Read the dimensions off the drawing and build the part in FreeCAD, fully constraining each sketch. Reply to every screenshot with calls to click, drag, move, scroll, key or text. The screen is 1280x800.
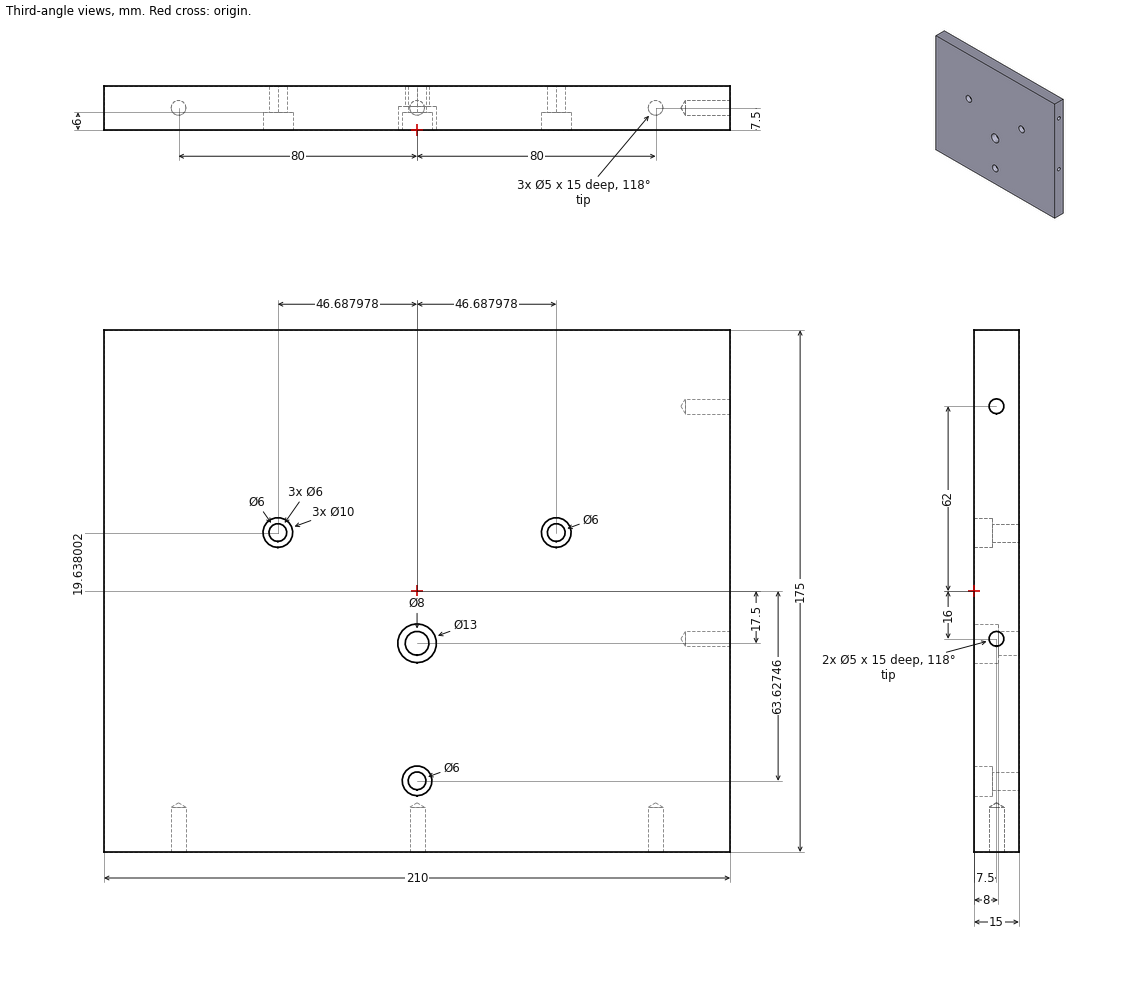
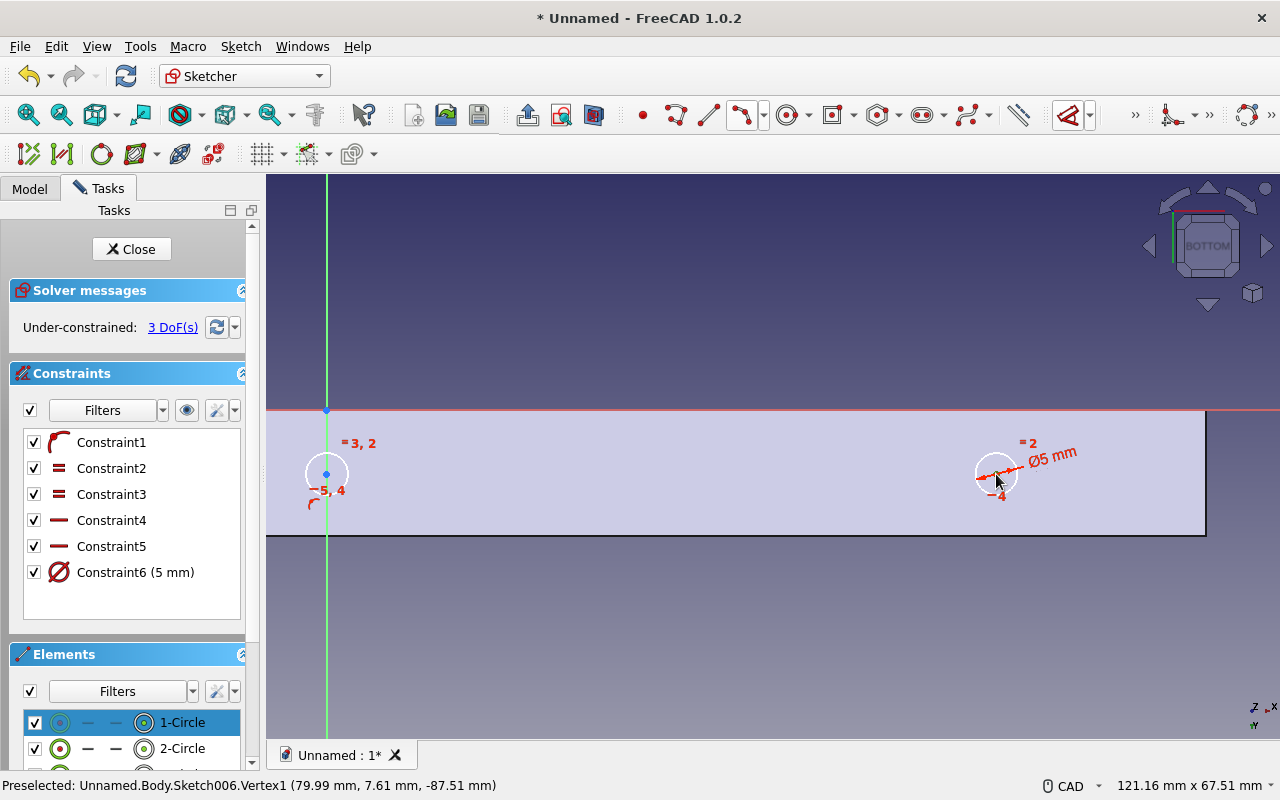
click(1090, 116)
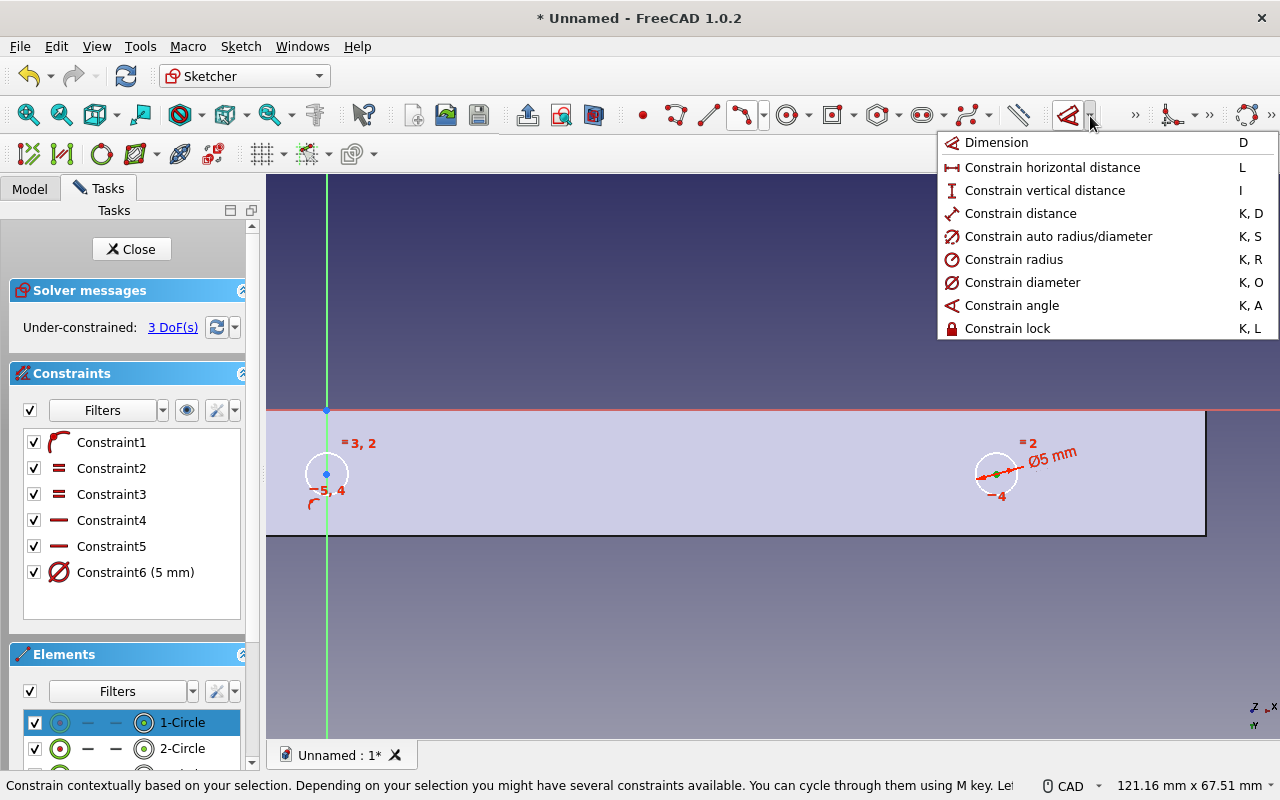
click(1108, 168)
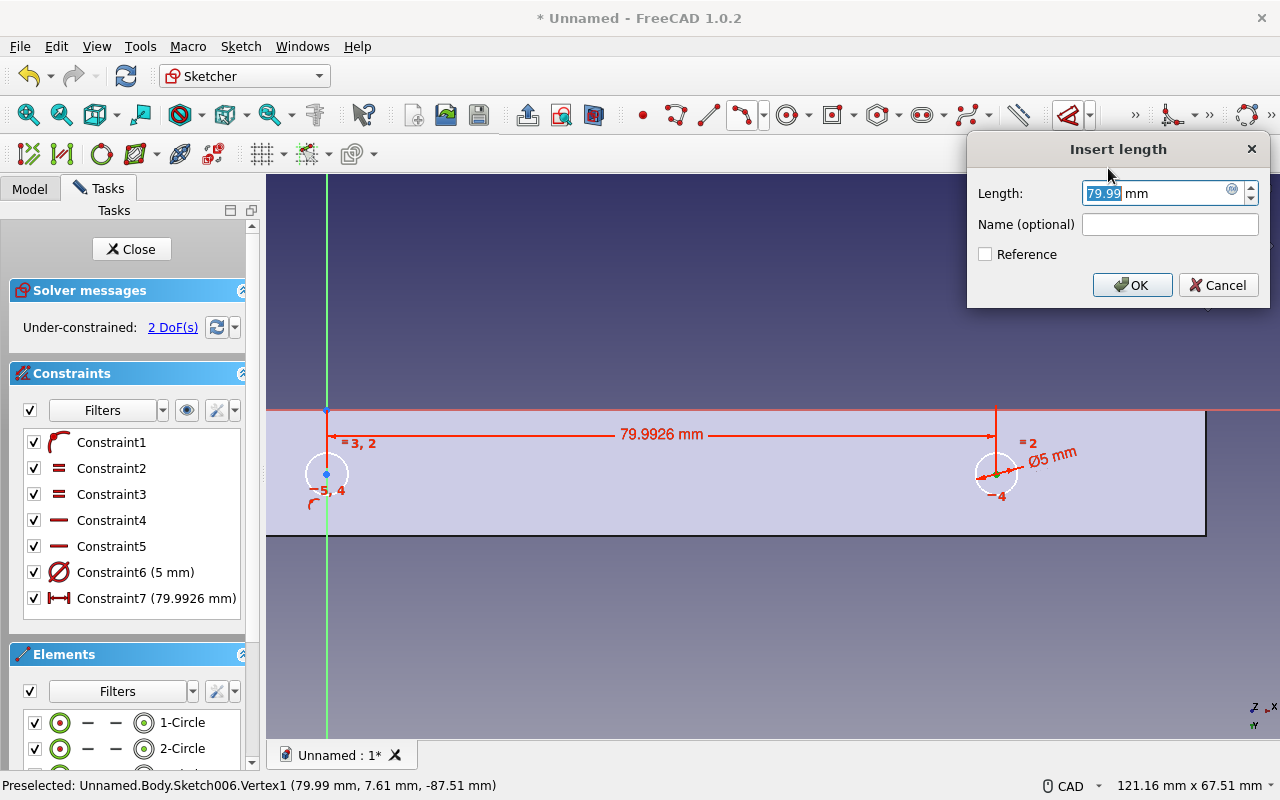
text(80)
key(Return)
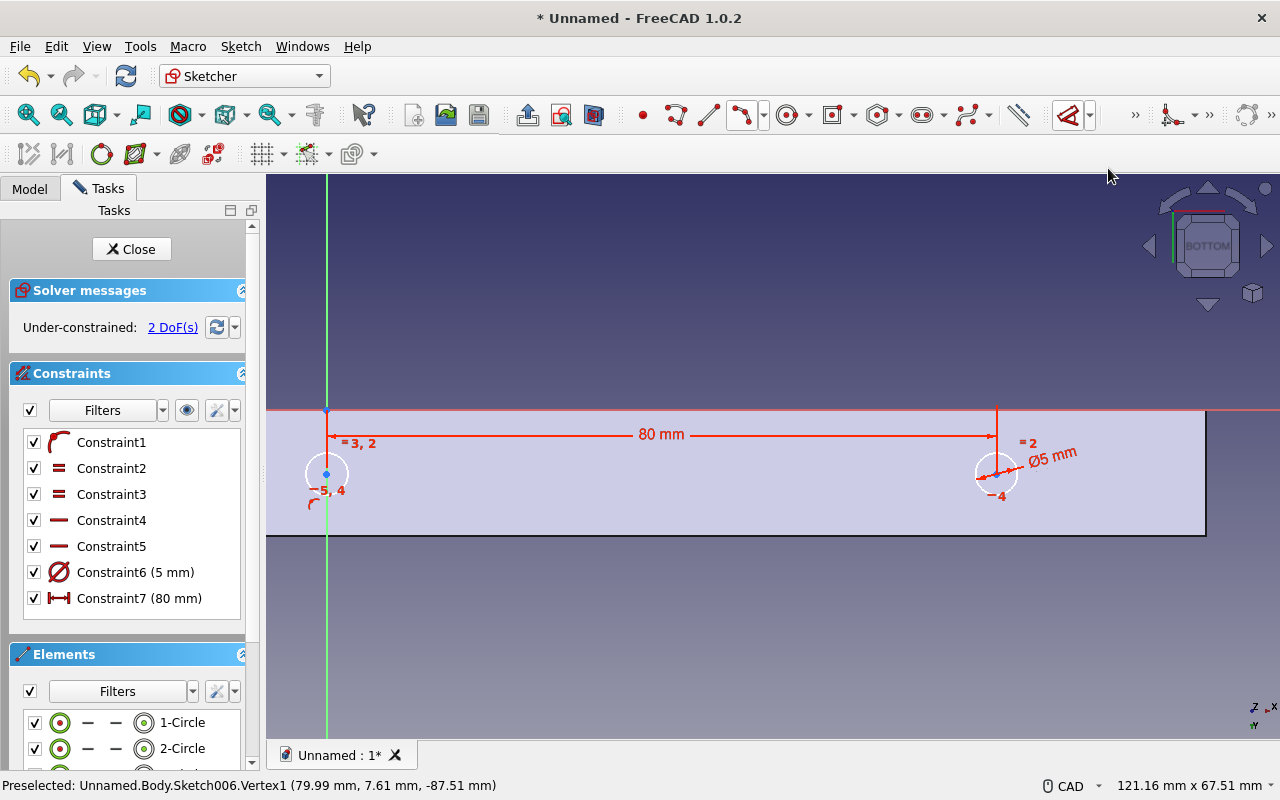
scroll(1013, 460, down, 4)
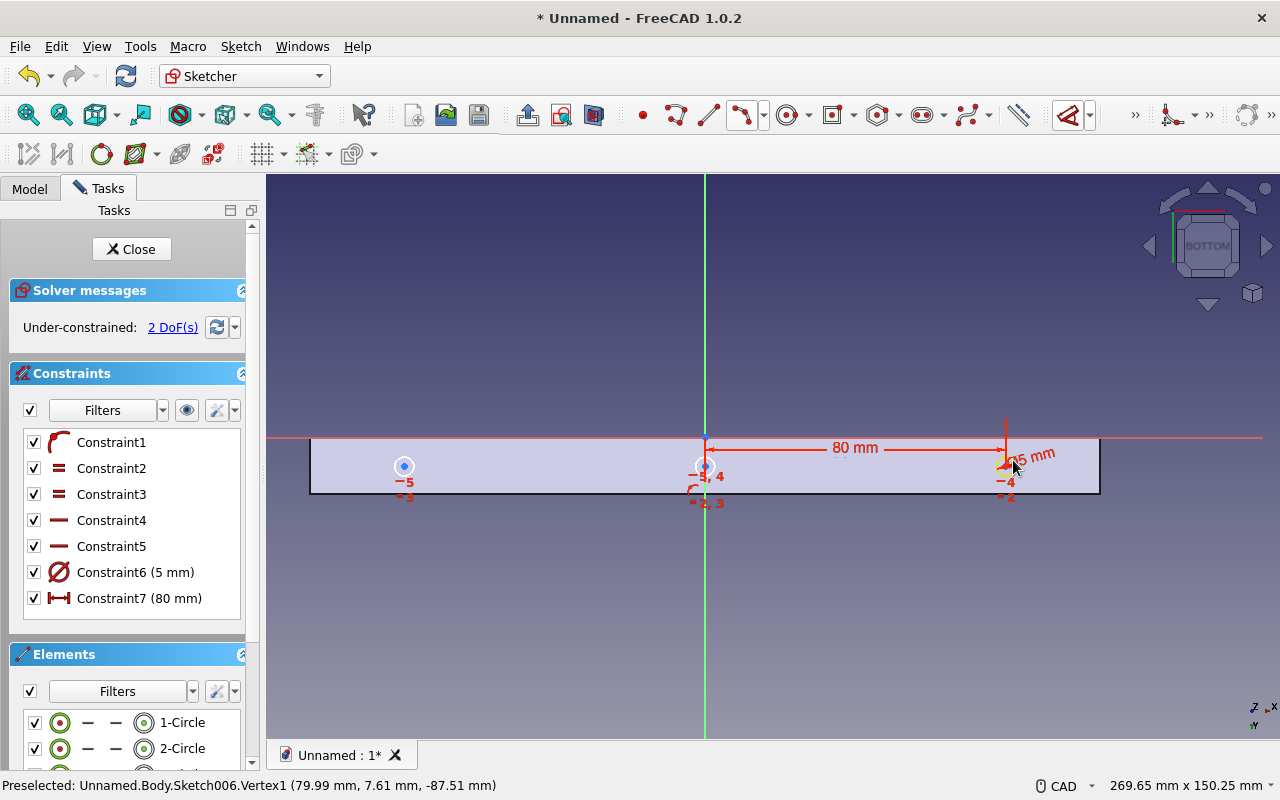
click(404, 467)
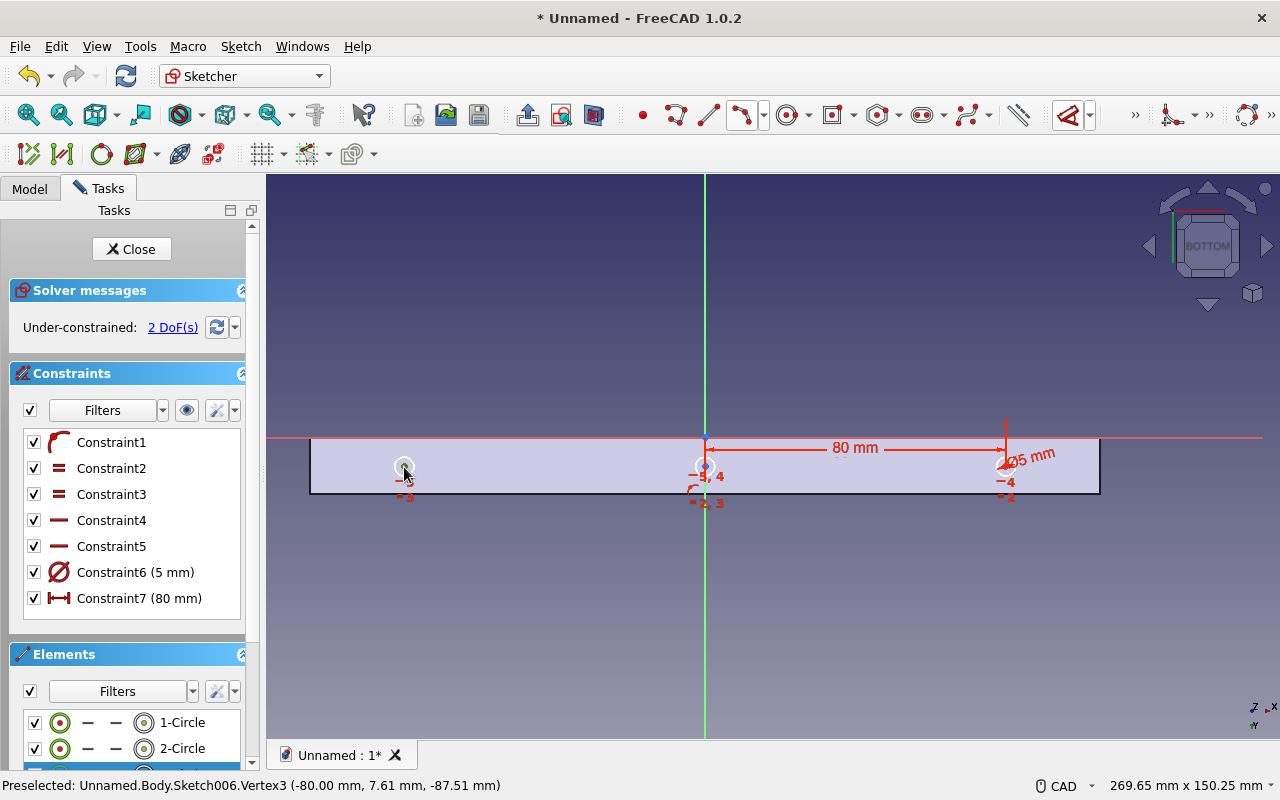
click(1090, 116)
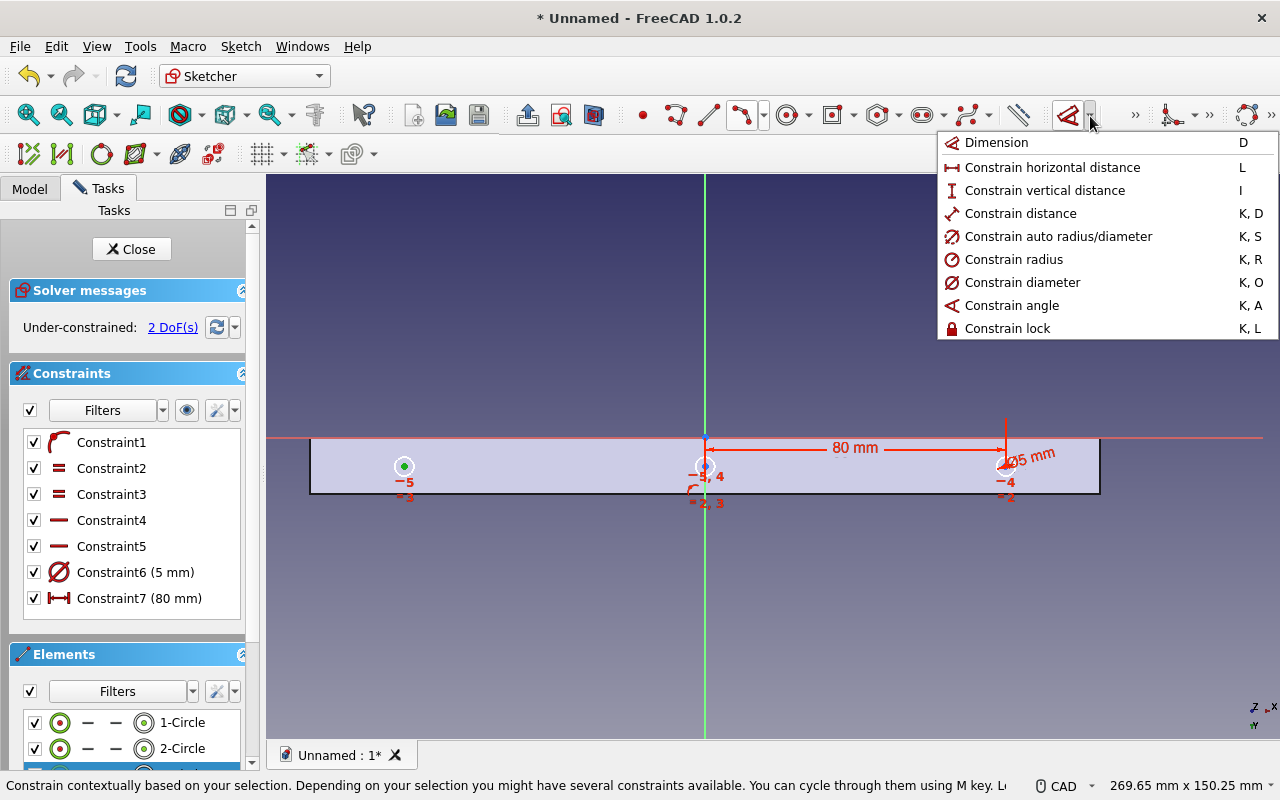
click(1108, 168)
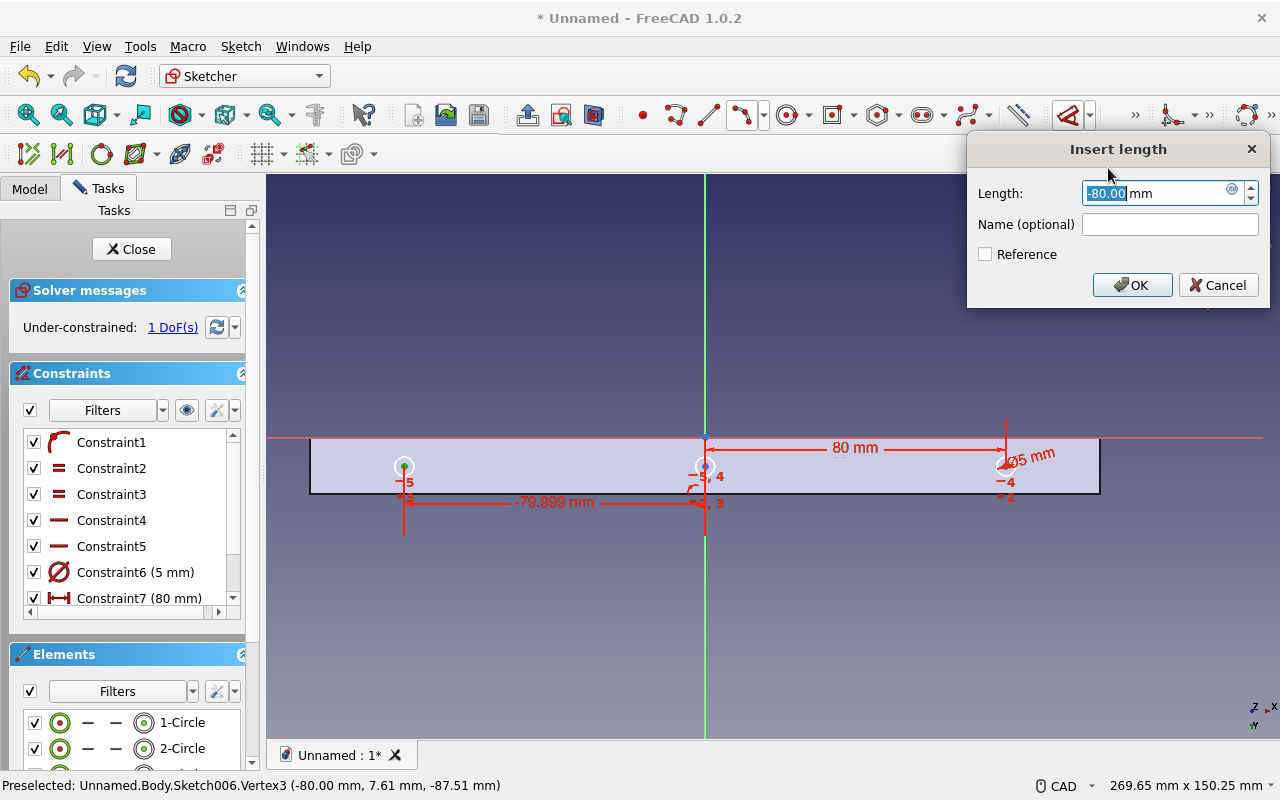
text(-80)
key(Return)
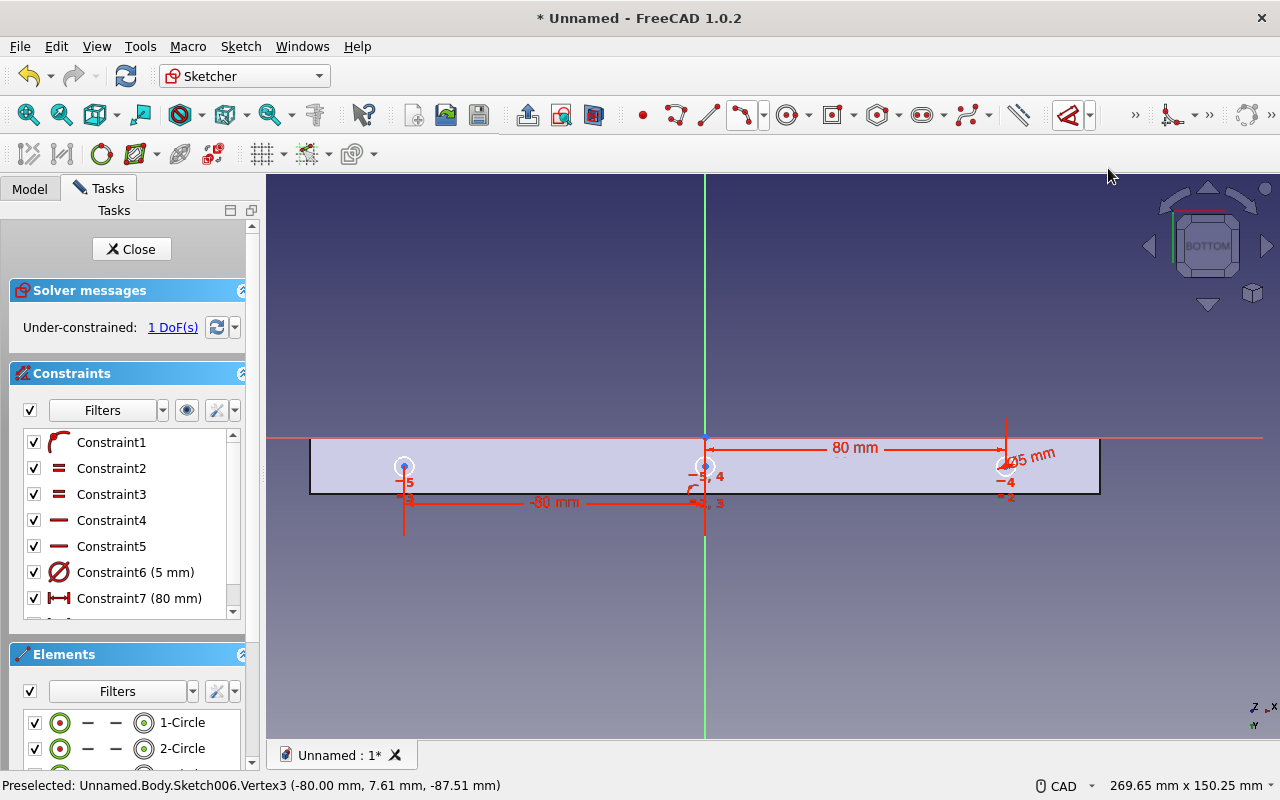
scroll(1006, 467, up, 2)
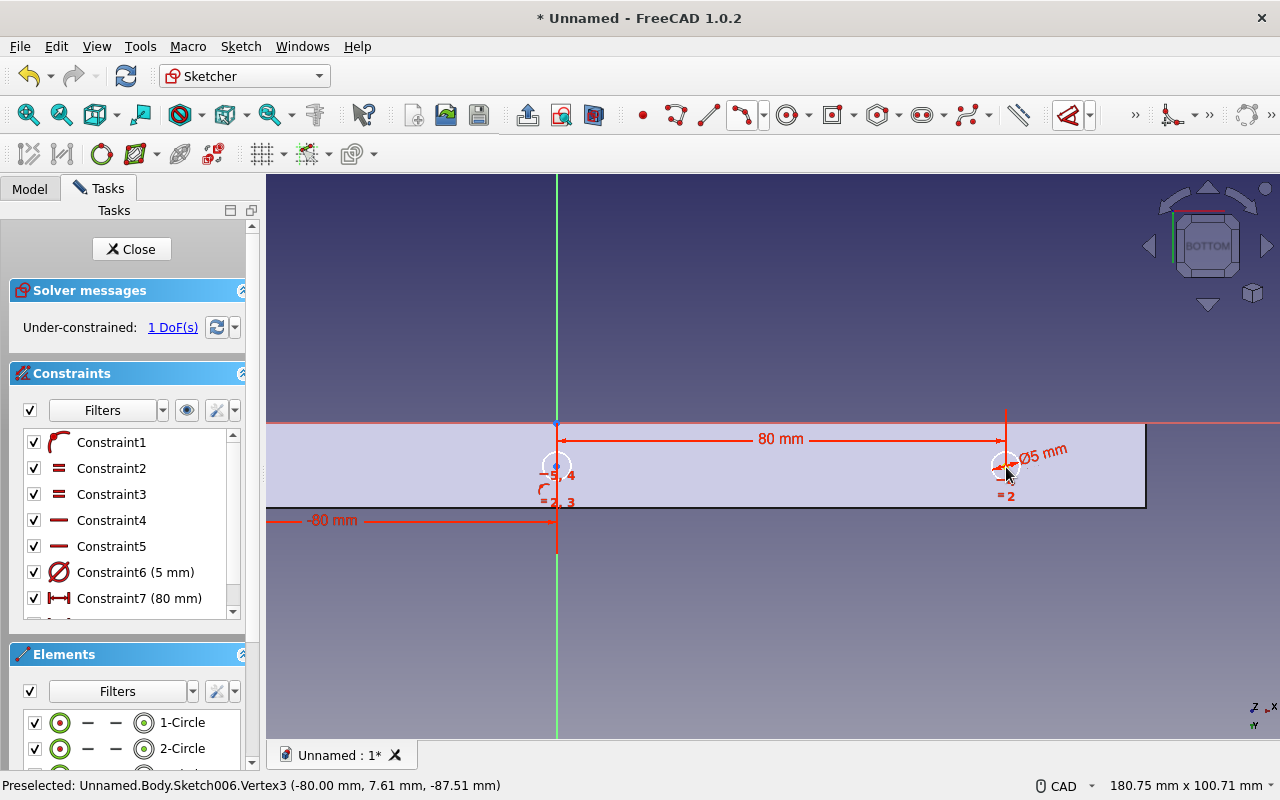
click(1006, 466)